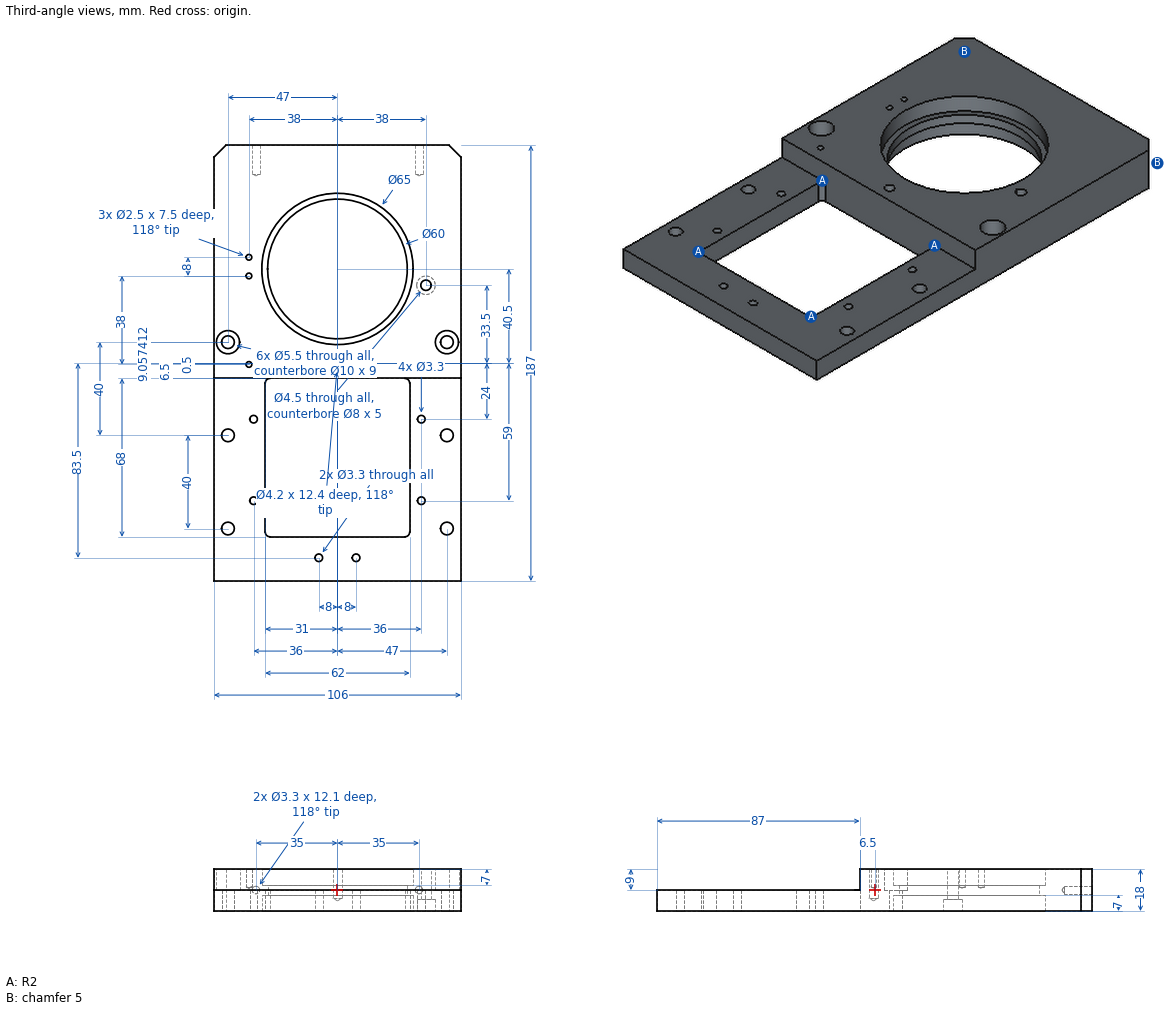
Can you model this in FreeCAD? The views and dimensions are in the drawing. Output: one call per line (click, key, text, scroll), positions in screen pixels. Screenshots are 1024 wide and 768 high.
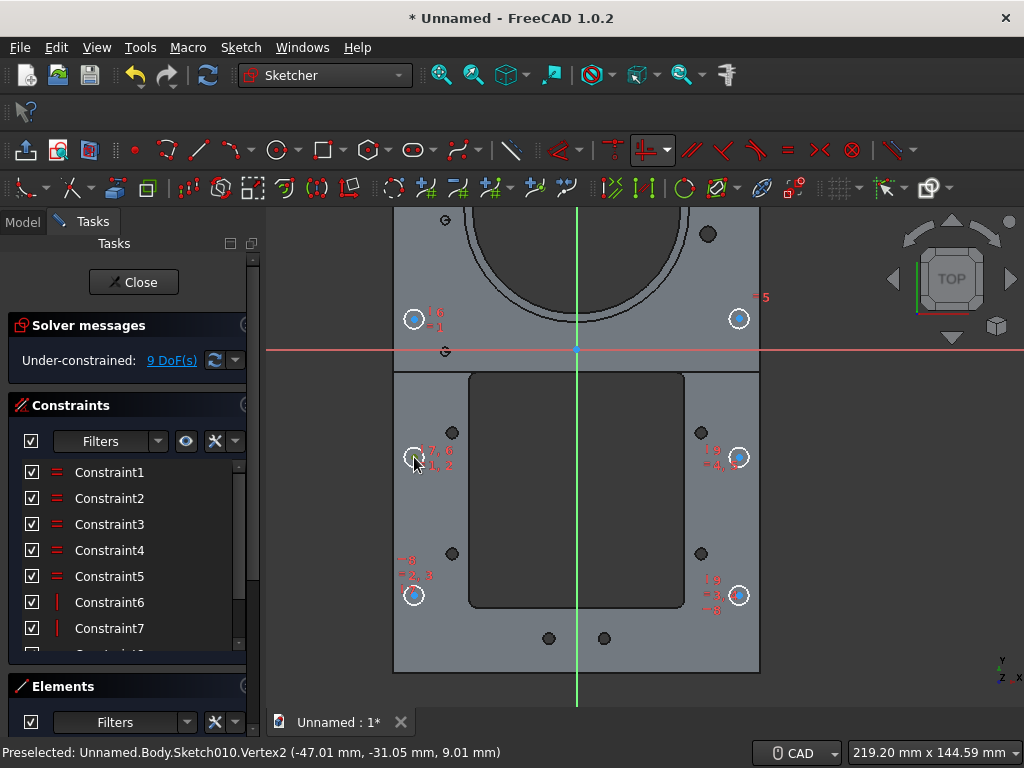
click(739, 457)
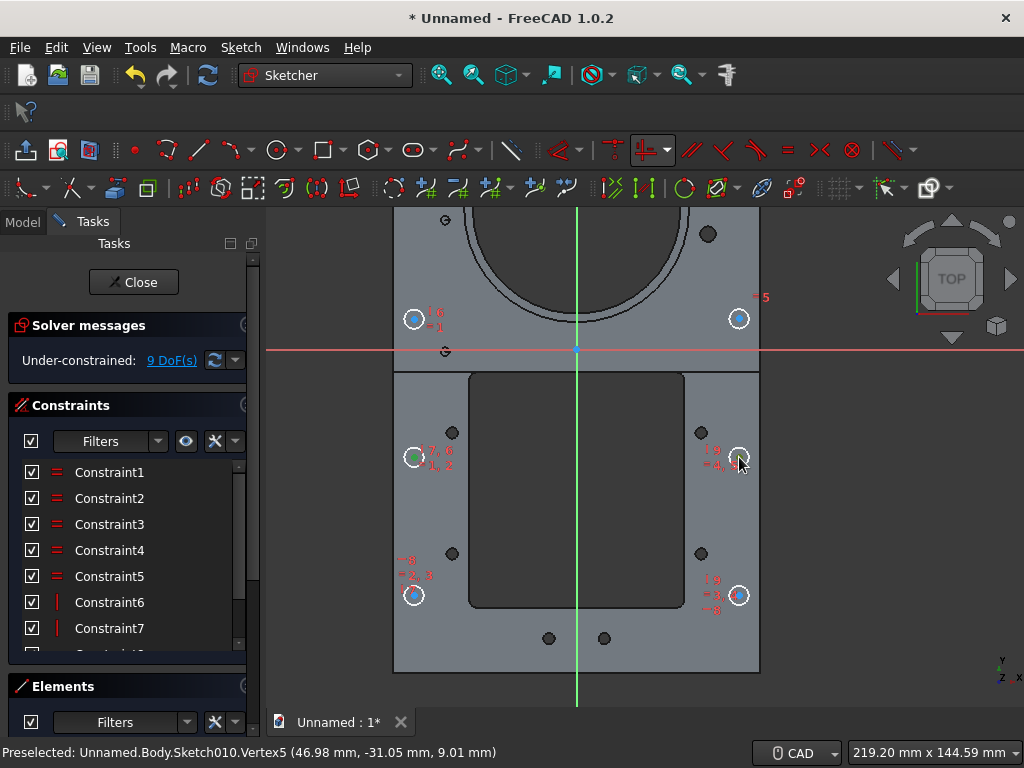
key(h)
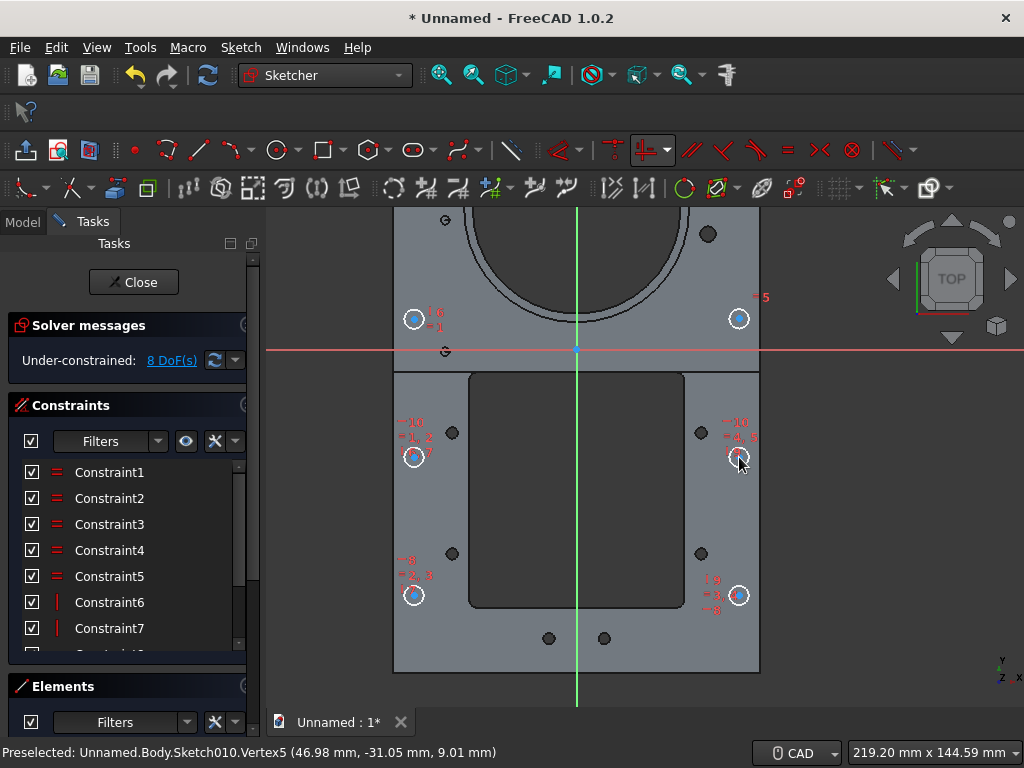
click(737, 459)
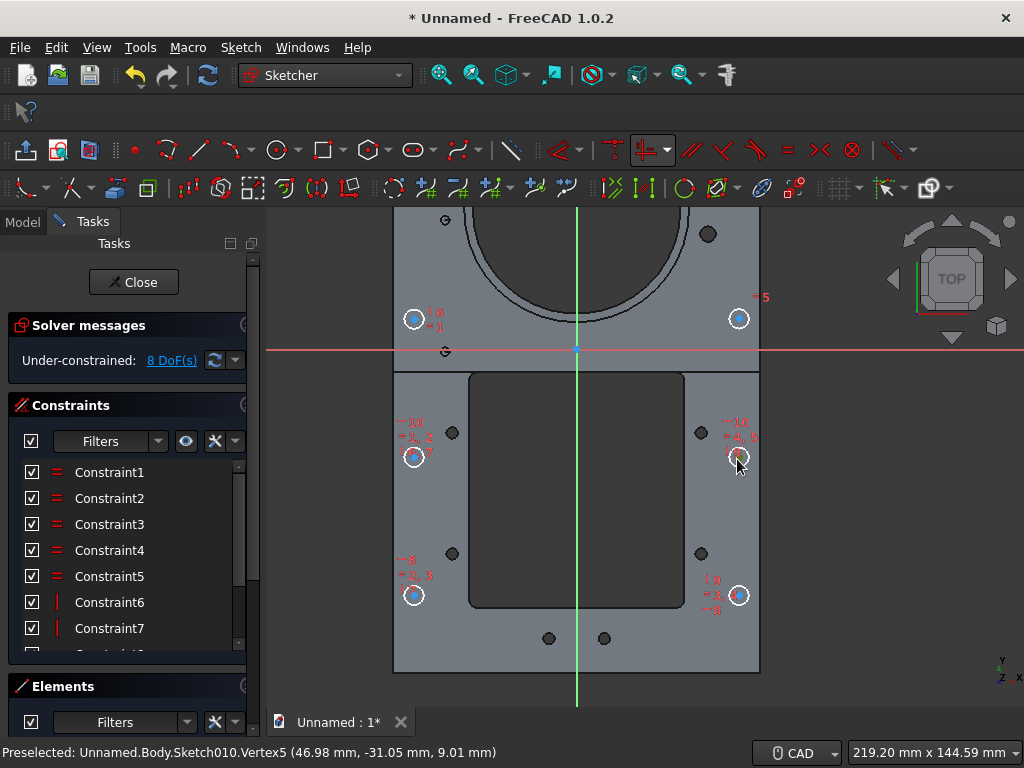
click(739, 319)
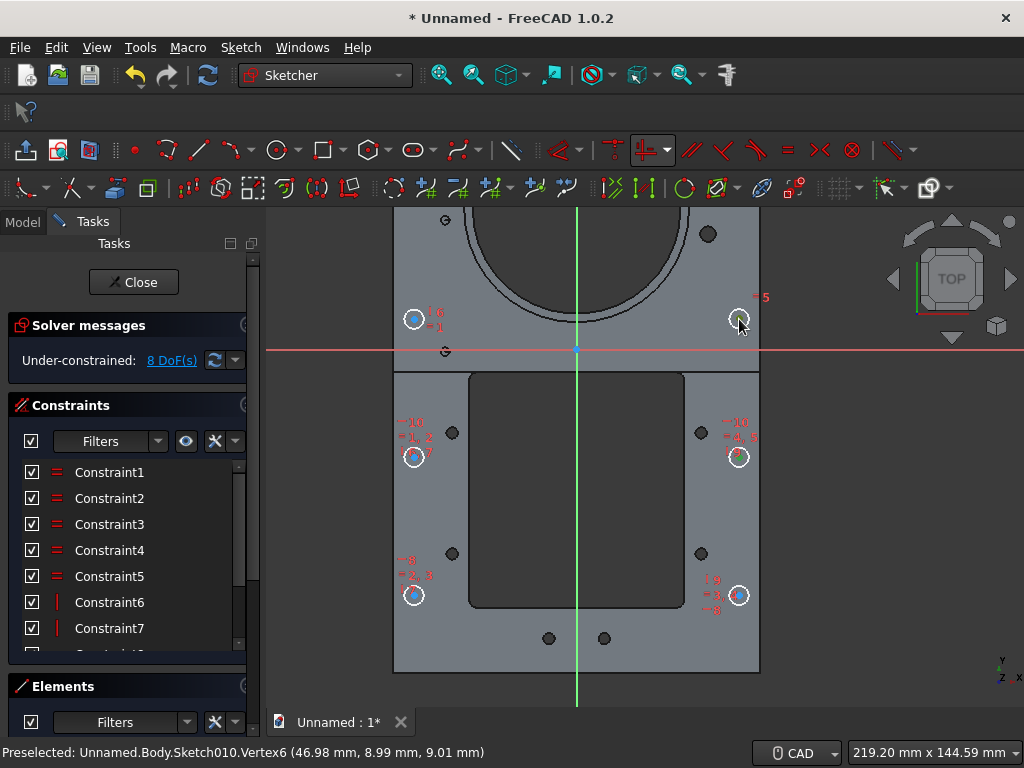
click(670, 150)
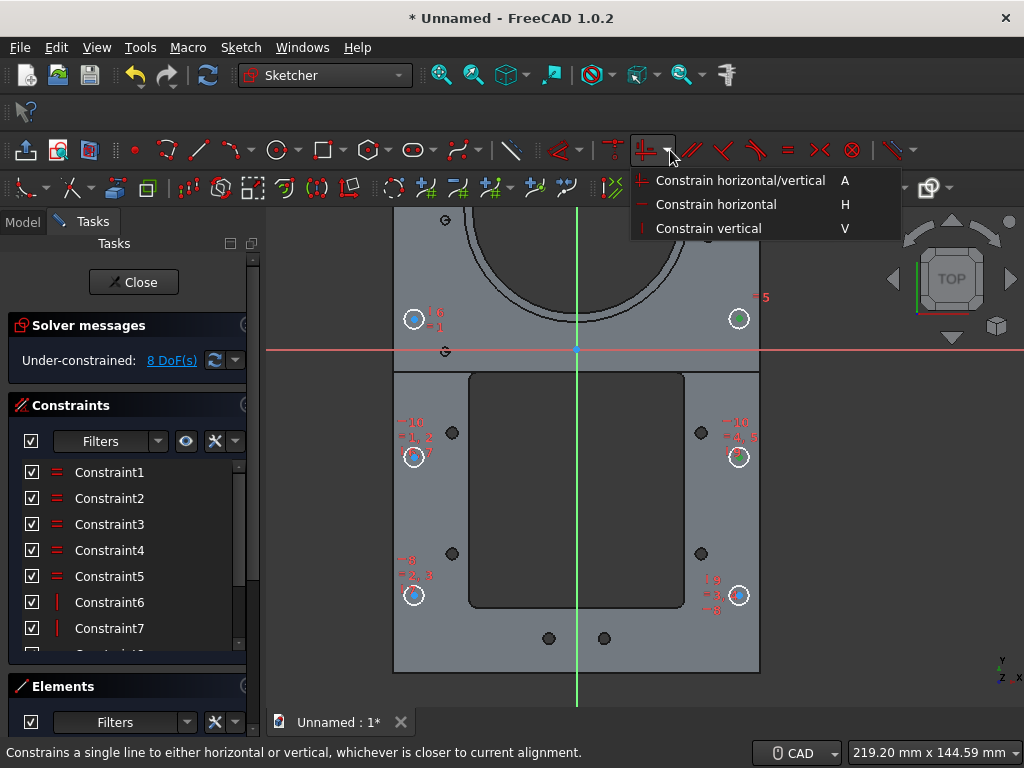
click(766, 228)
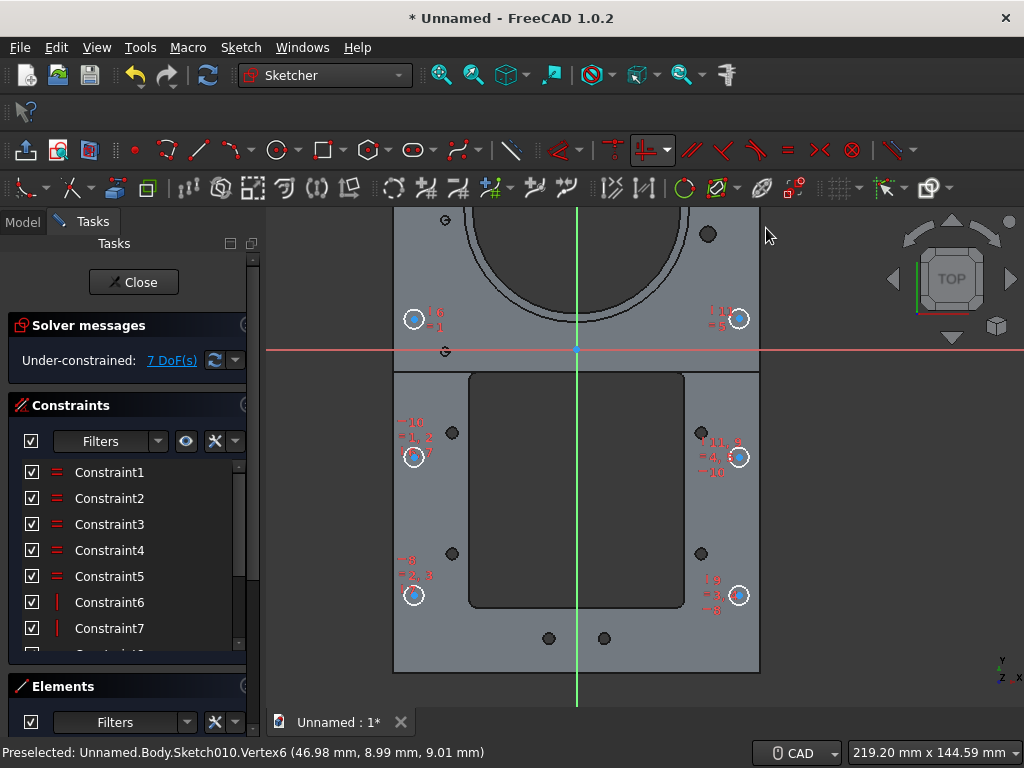
click(414, 319)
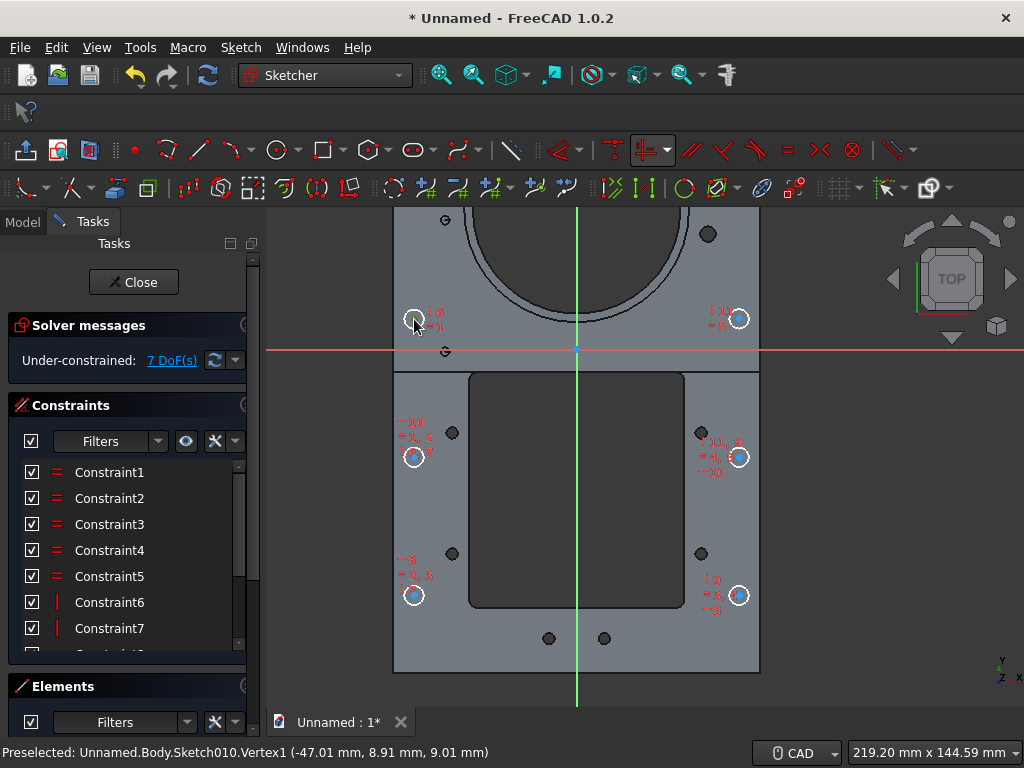
click(739, 319)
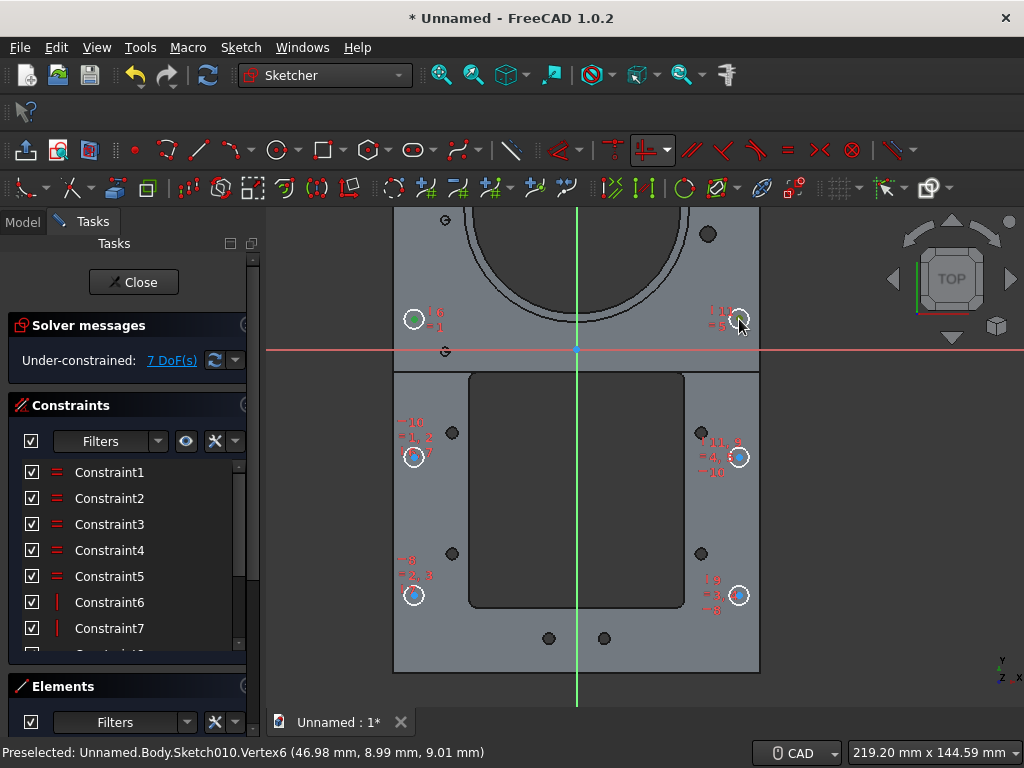
click(670, 150)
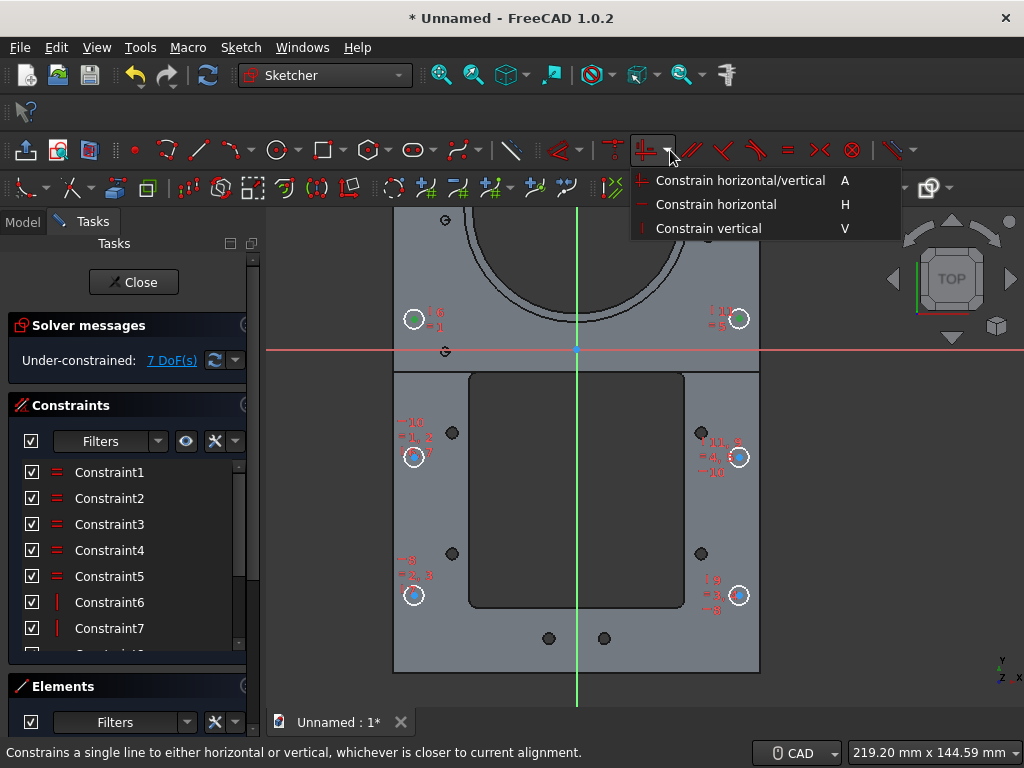
click(766, 204)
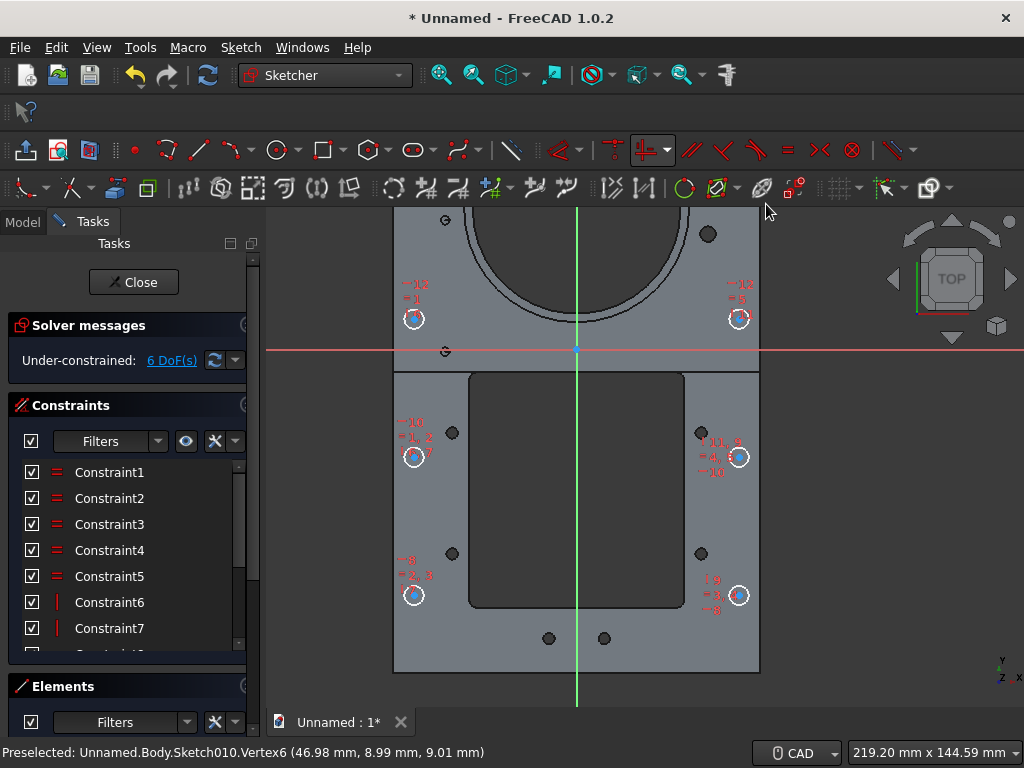
click(558, 150)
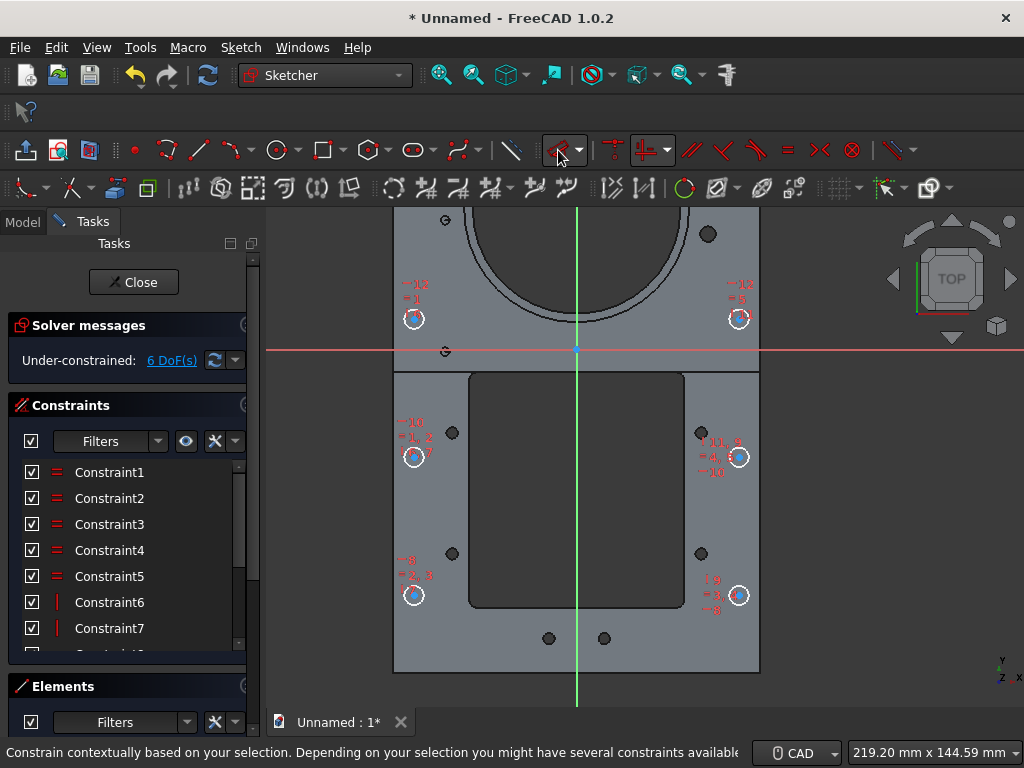
scroll(421, 312, up, 4)